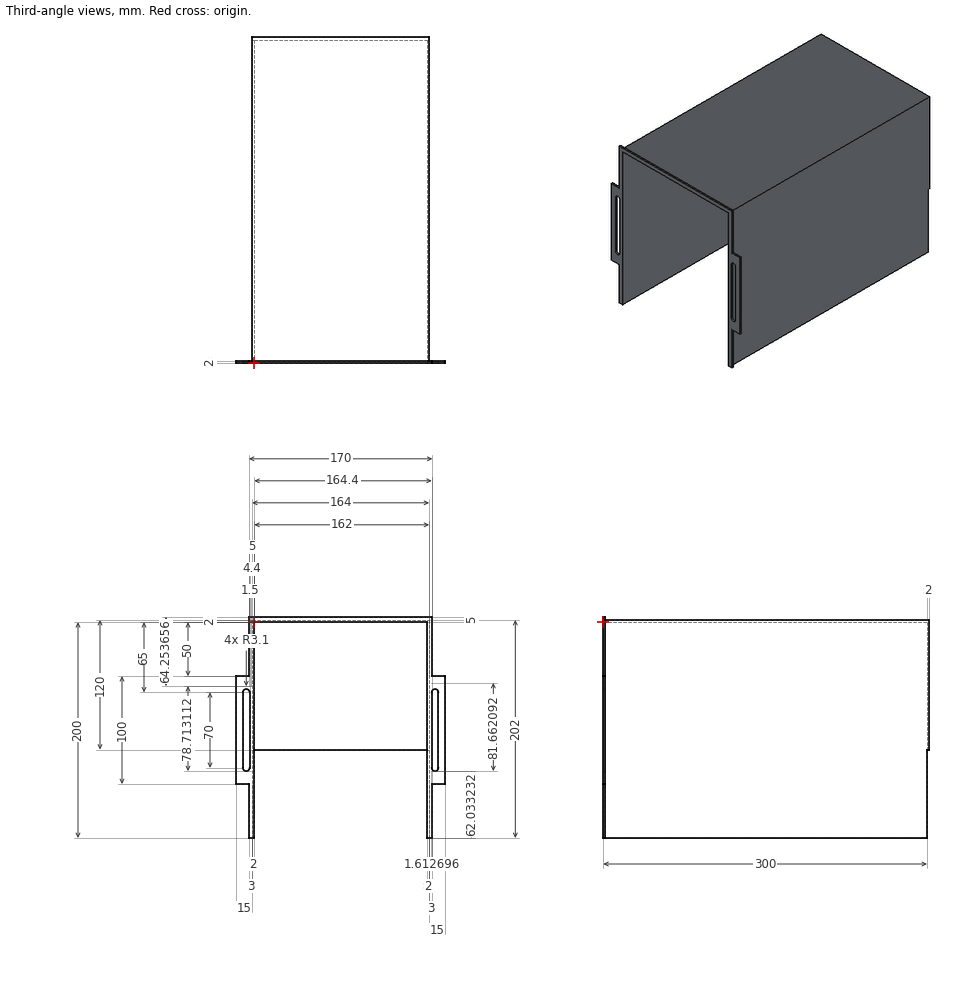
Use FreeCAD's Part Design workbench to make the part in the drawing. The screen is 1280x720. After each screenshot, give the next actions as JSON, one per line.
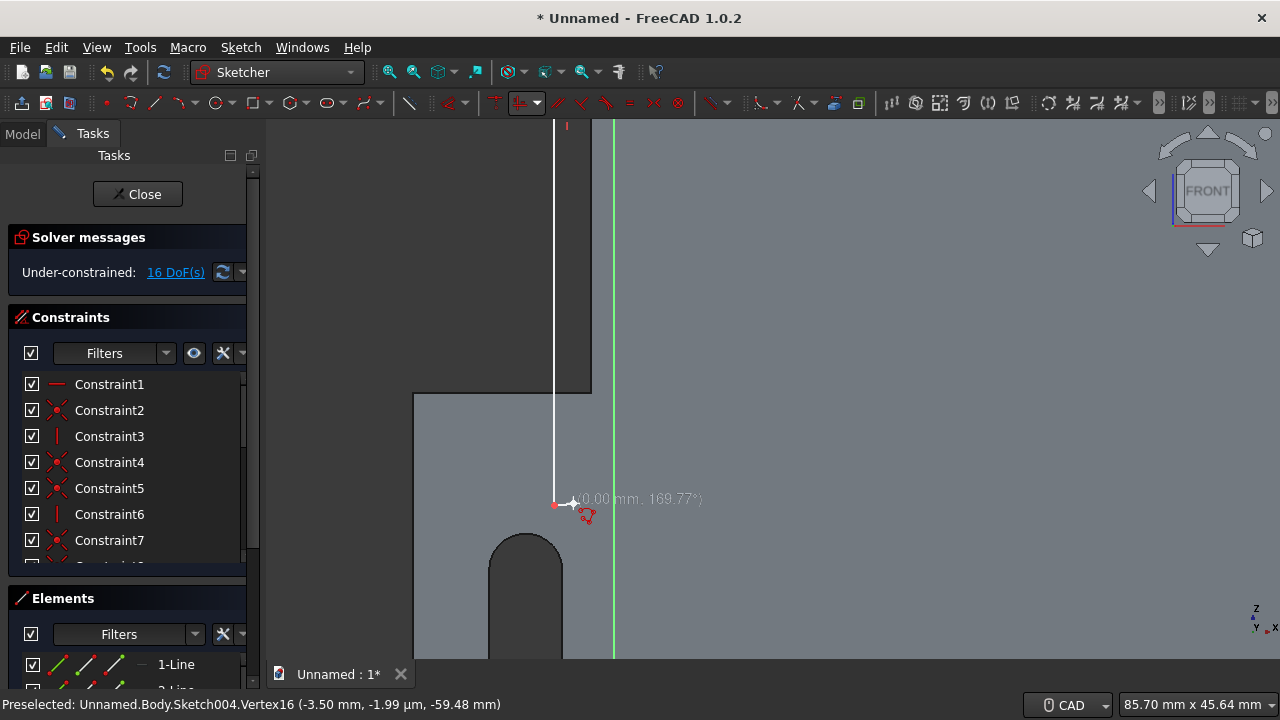
{"action": "scroll", "coordinate": [570, 300], "scroll_direction": "down", "scroll_amount": 10}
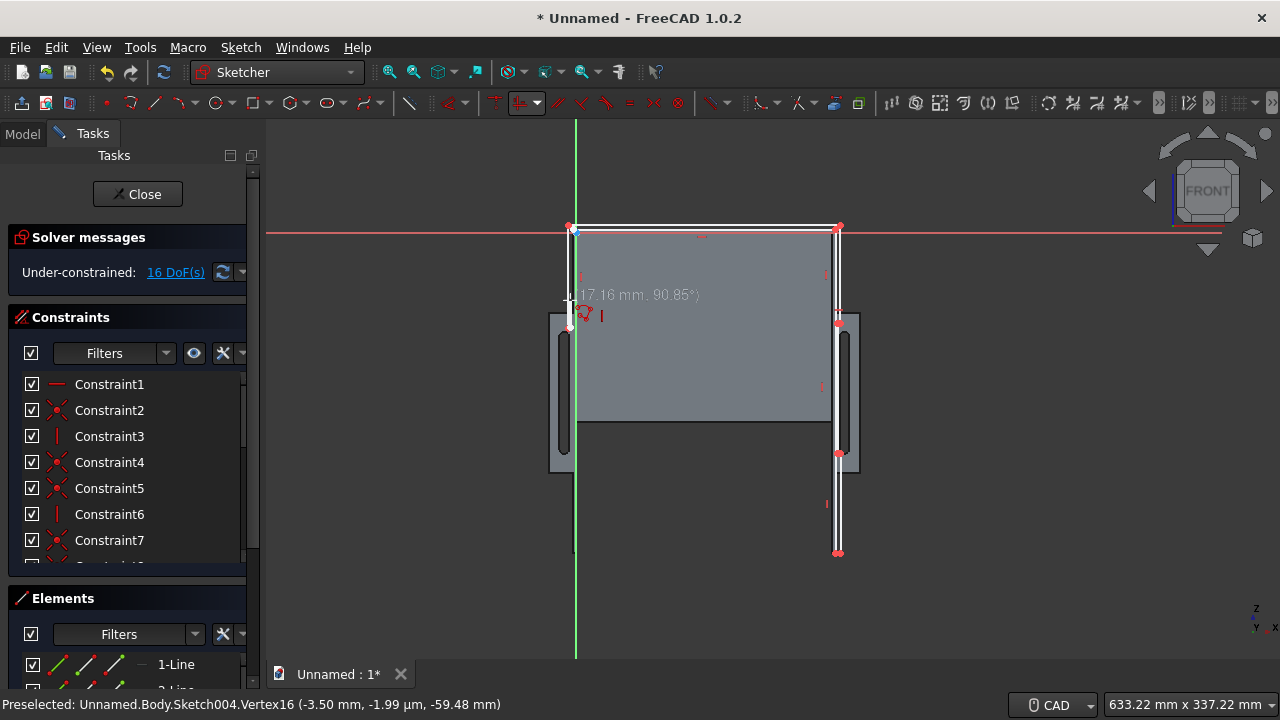
{"action": "scroll", "coordinate": [571, 454], "scroll_direction": "up", "scroll_amount": 6}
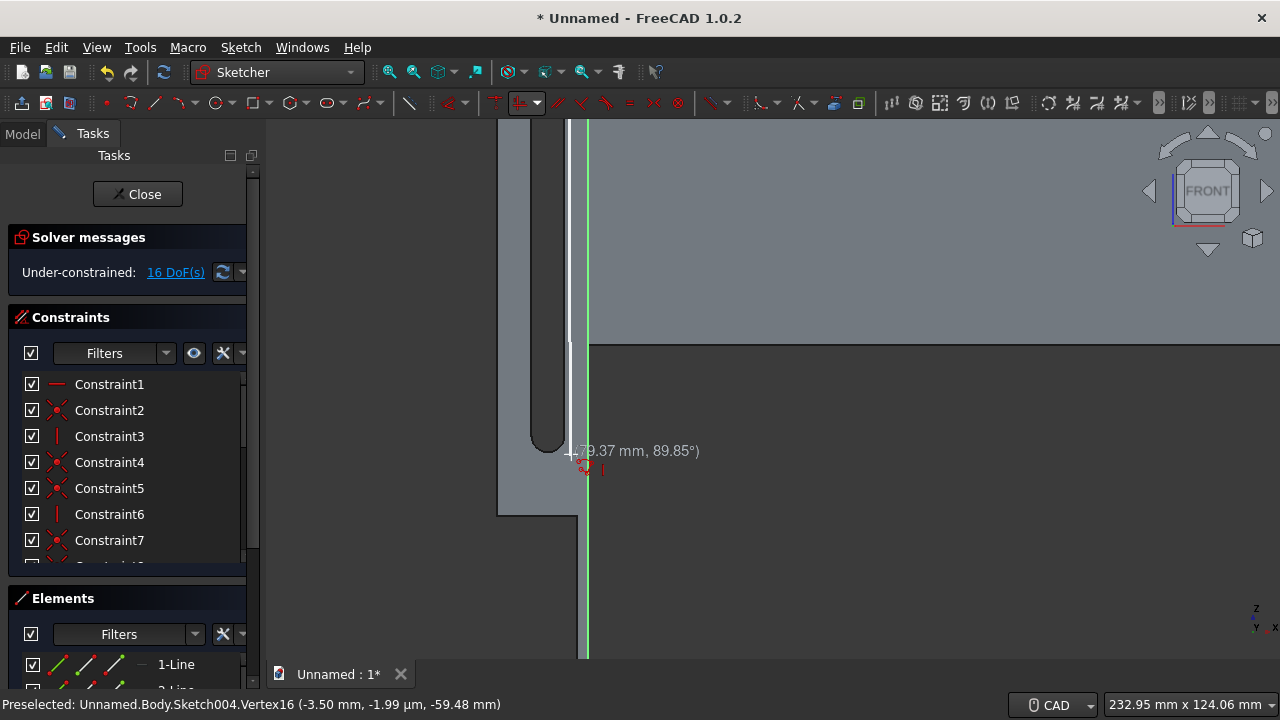
{"action": "left_click", "coordinate": [569, 452]}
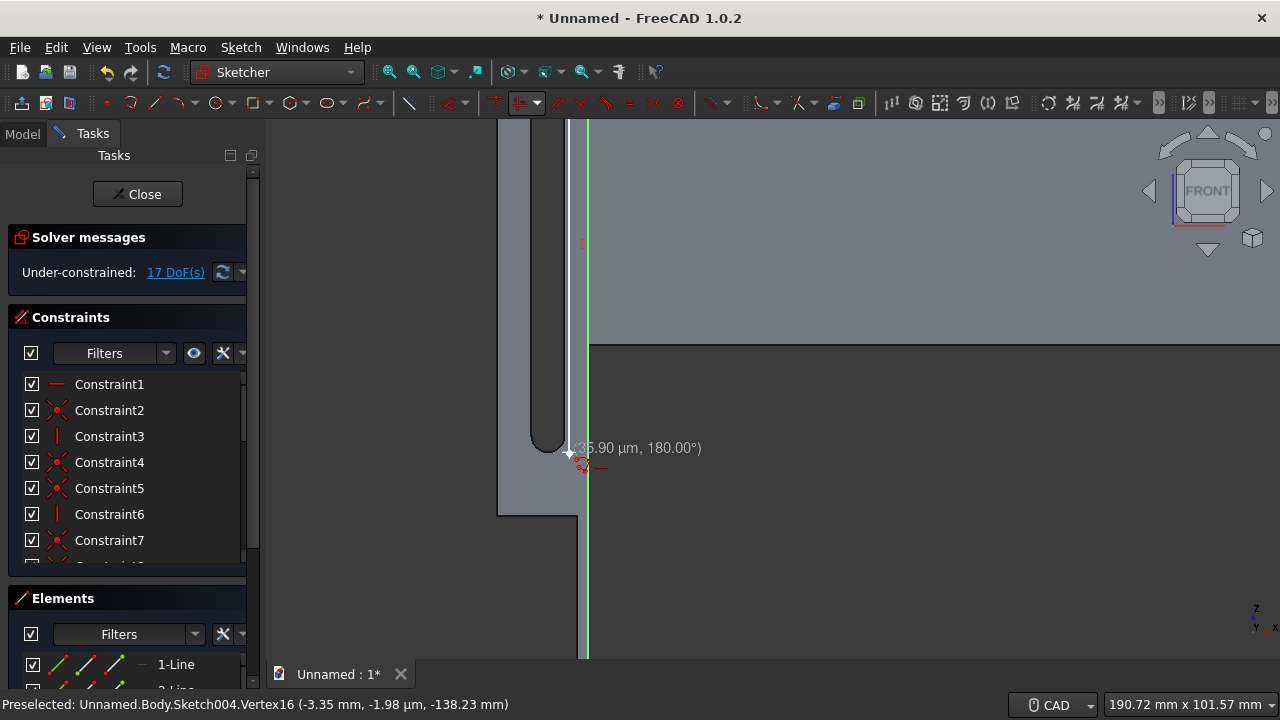
{"action": "scroll", "coordinate": [561, 452], "scroll_direction": "up", "scroll_amount": 4}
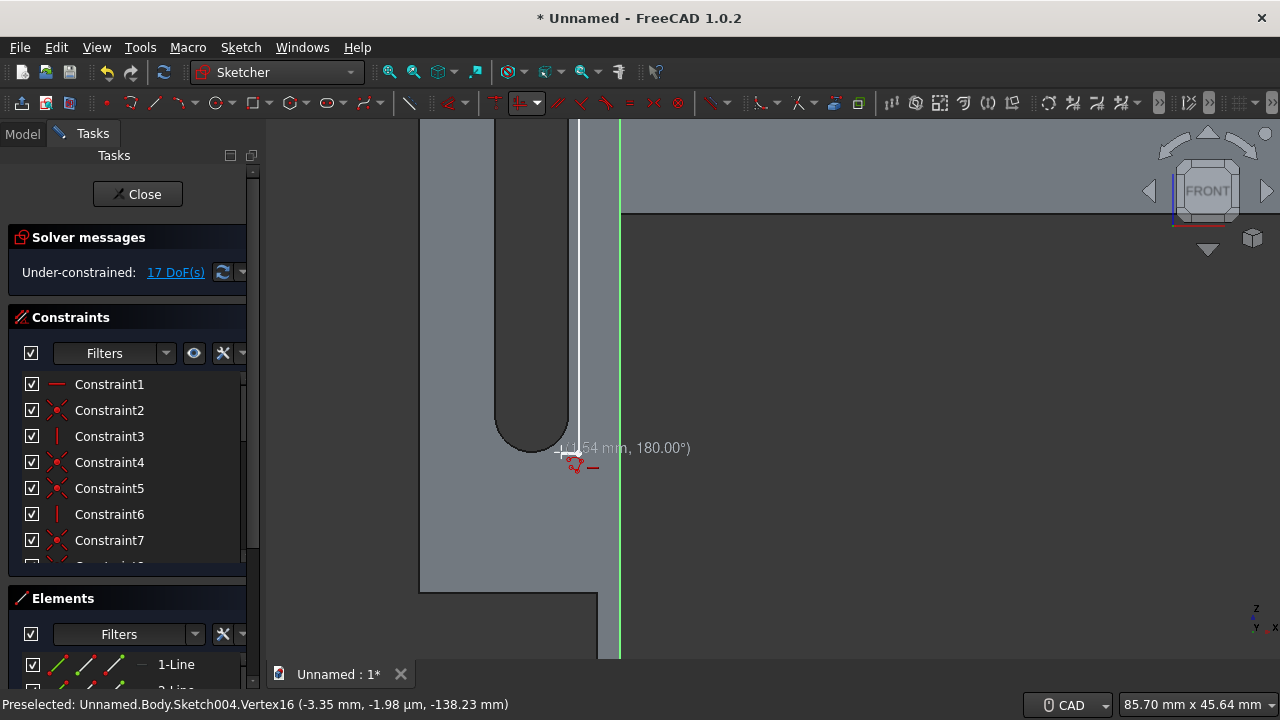
{"action": "left_click", "coordinate": [561, 451]}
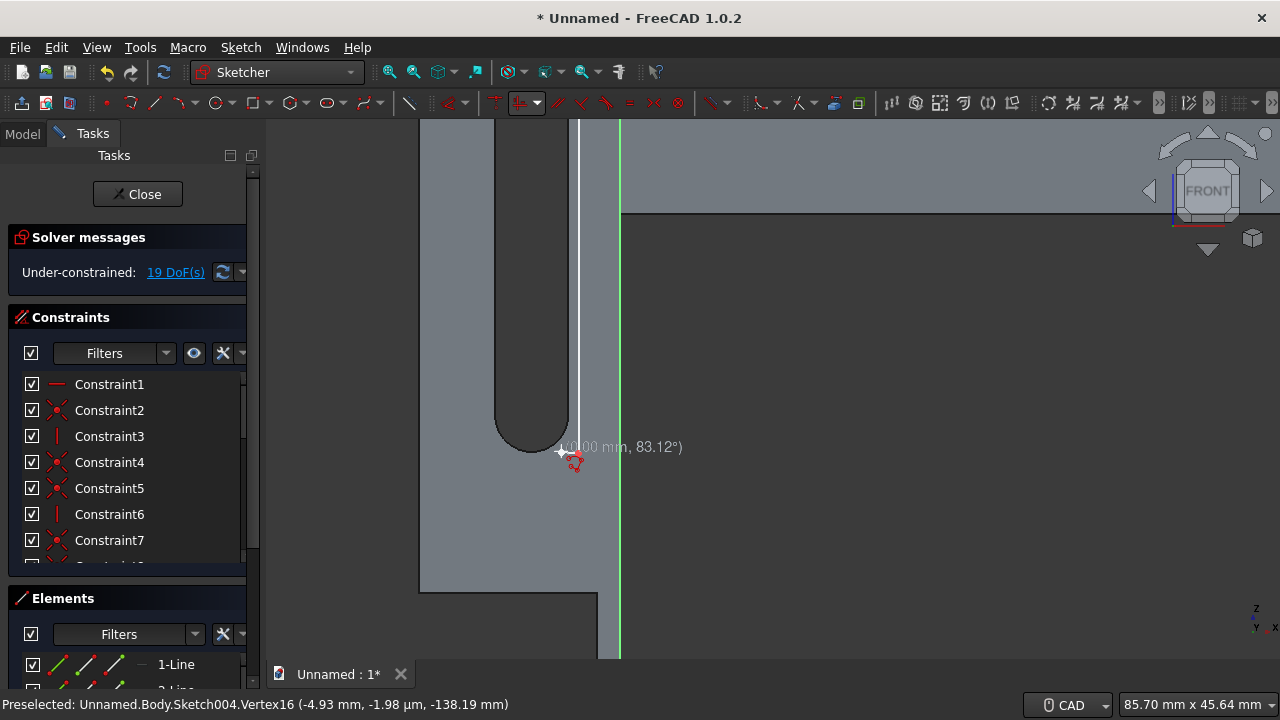
{"action": "scroll", "coordinate": [570, 454], "scroll_direction": "down", "scroll_amount": 10}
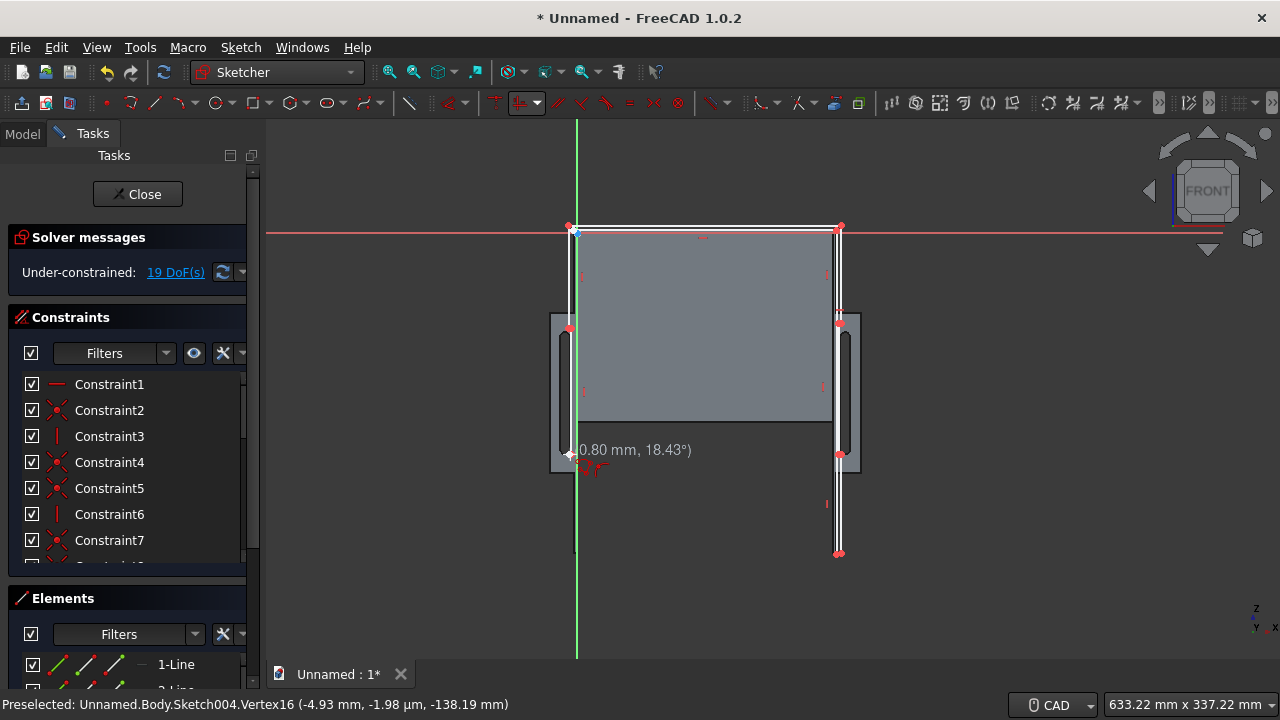
{"action": "scroll", "coordinate": [569, 553], "scroll_direction": "up", "scroll_amount": 4}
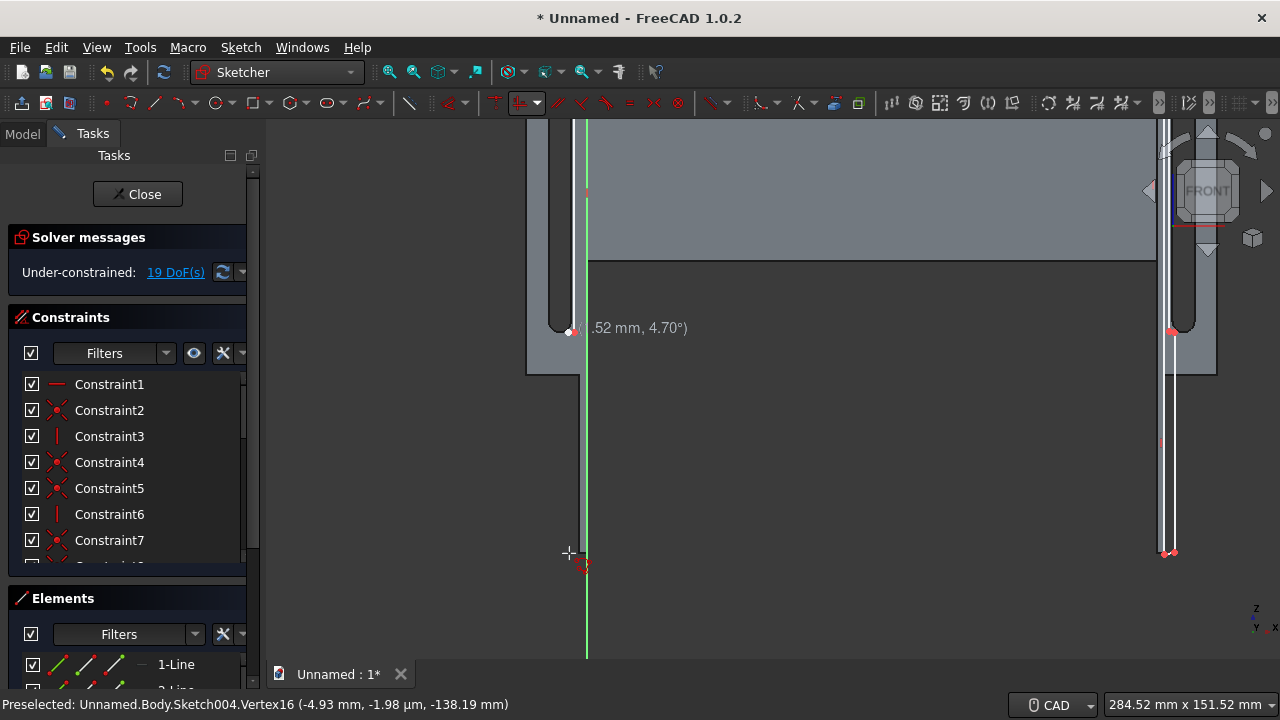
{"action": "left_click", "coordinate": [569, 553]}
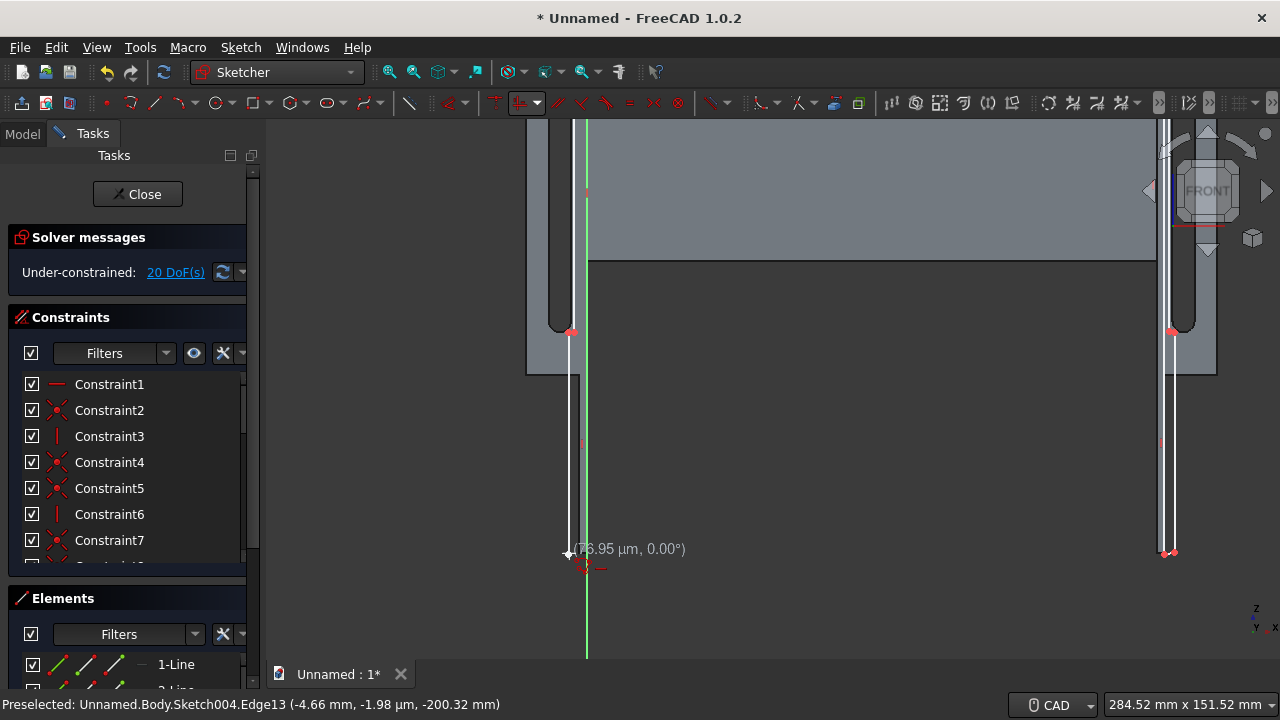
{"action": "scroll", "coordinate": [579, 553], "scroll_direction": "up", "scroll_amount": 5}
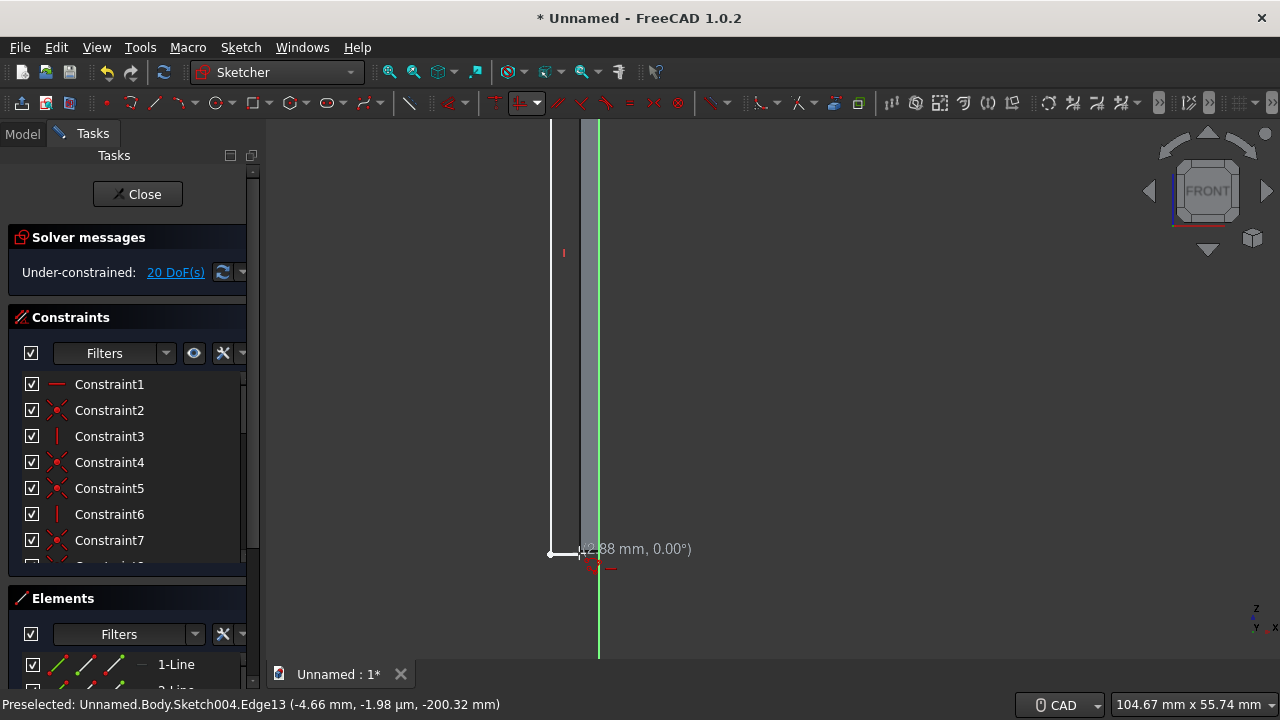
{"action": "left_click", "coordinate": [580, 552]}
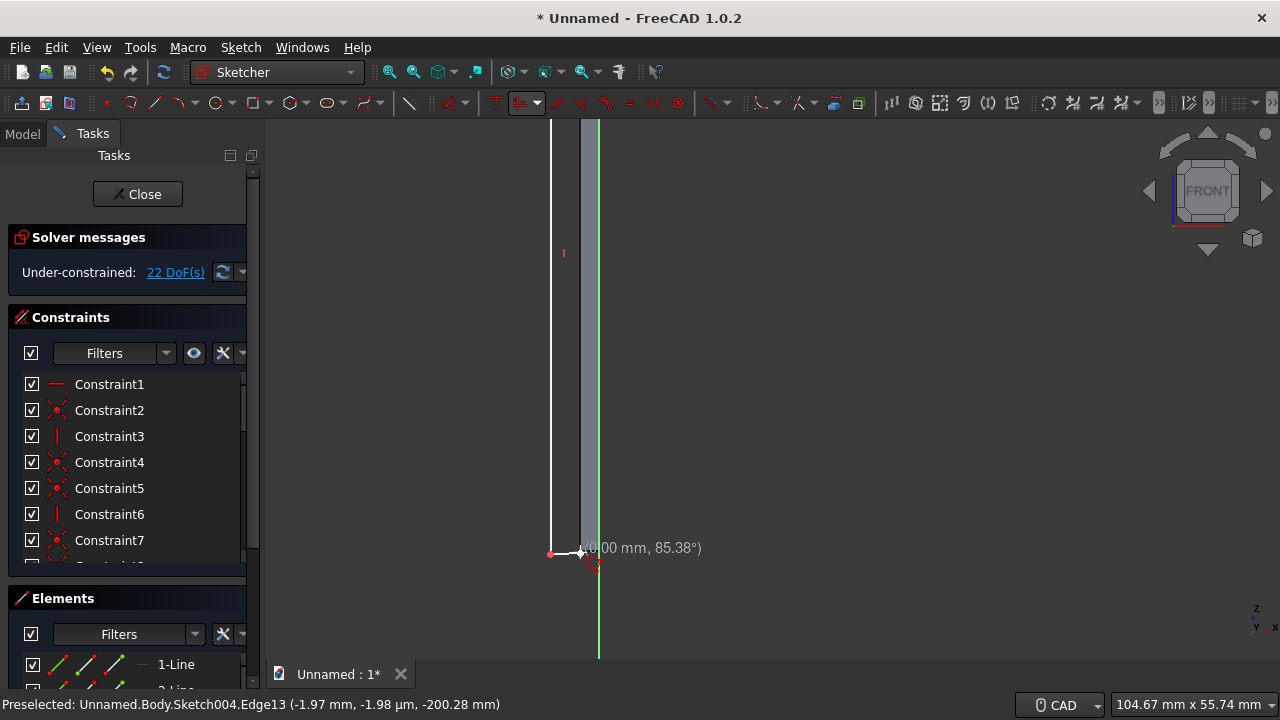
{"action": "scroll", "coordinate": [572, 554], "scroll_direction": "down", "scroll_amount": 9}